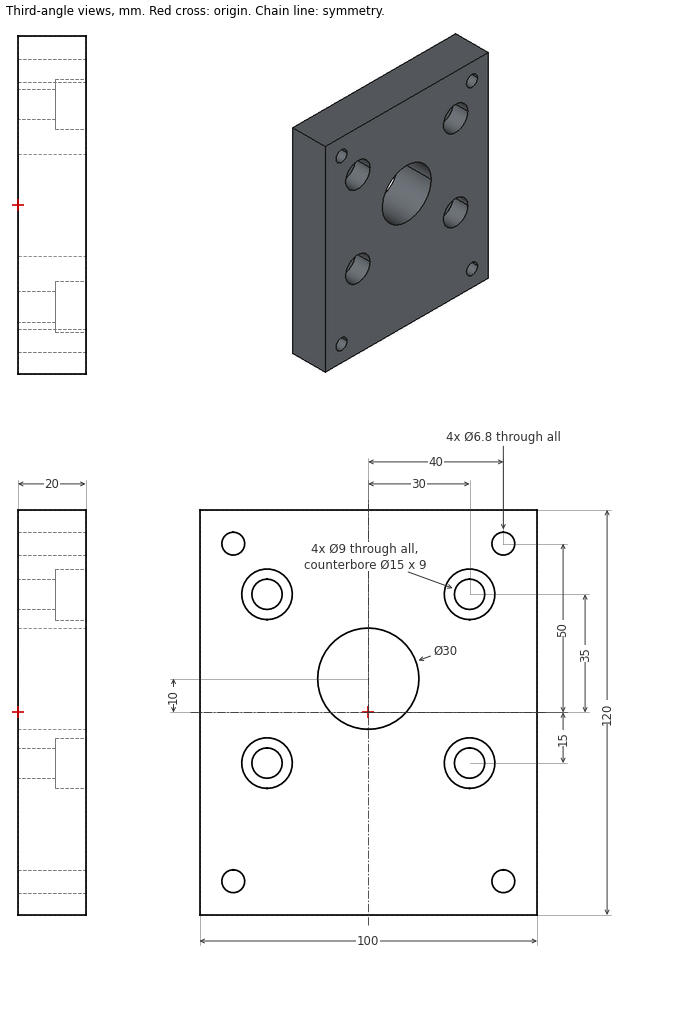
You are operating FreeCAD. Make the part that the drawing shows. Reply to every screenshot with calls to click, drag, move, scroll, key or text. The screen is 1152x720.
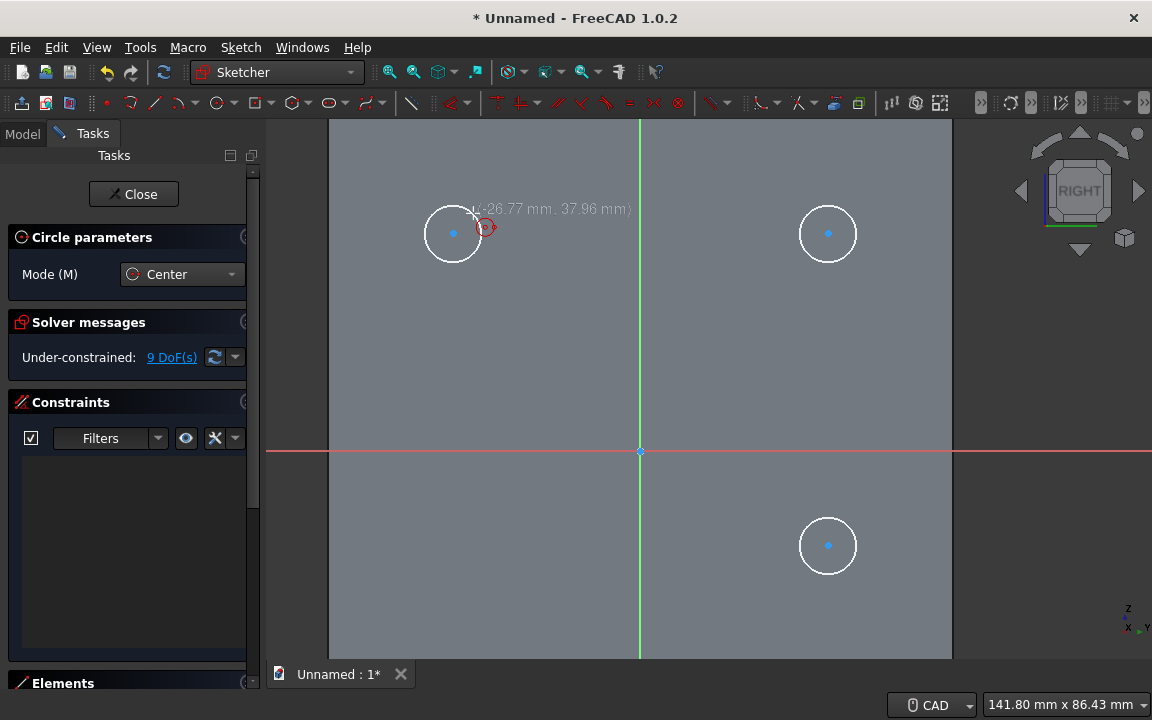
click(453, 545)
click(473, 525)
key(Escape)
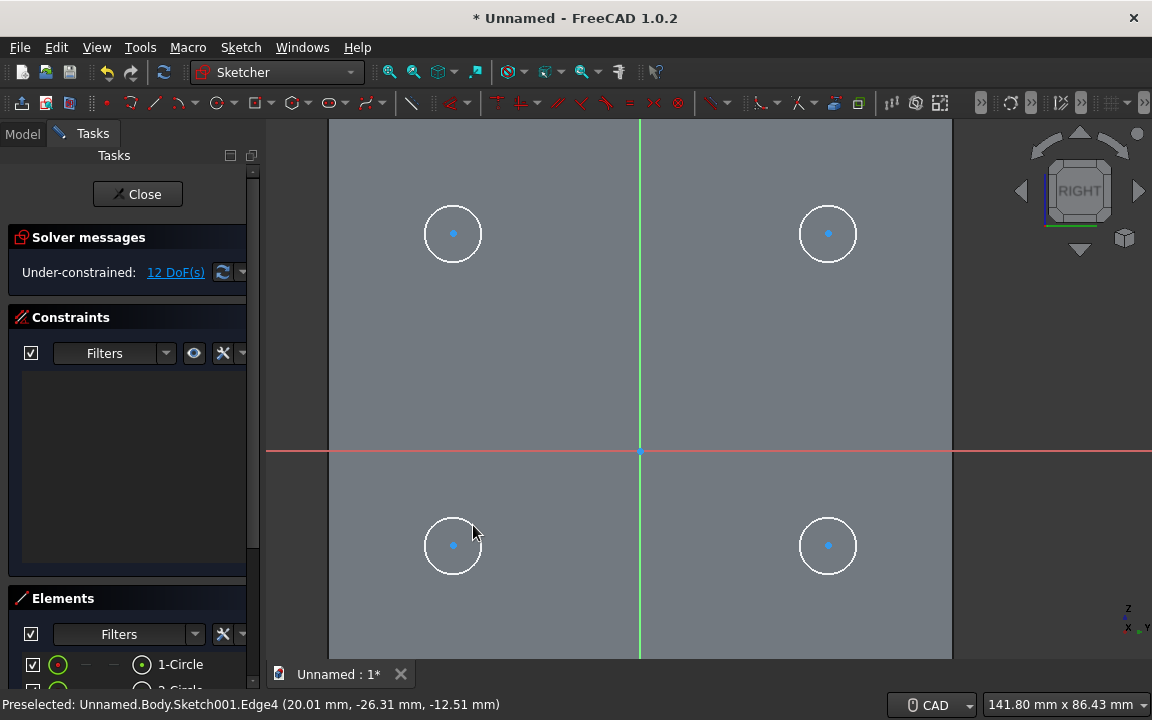
click(848, 214)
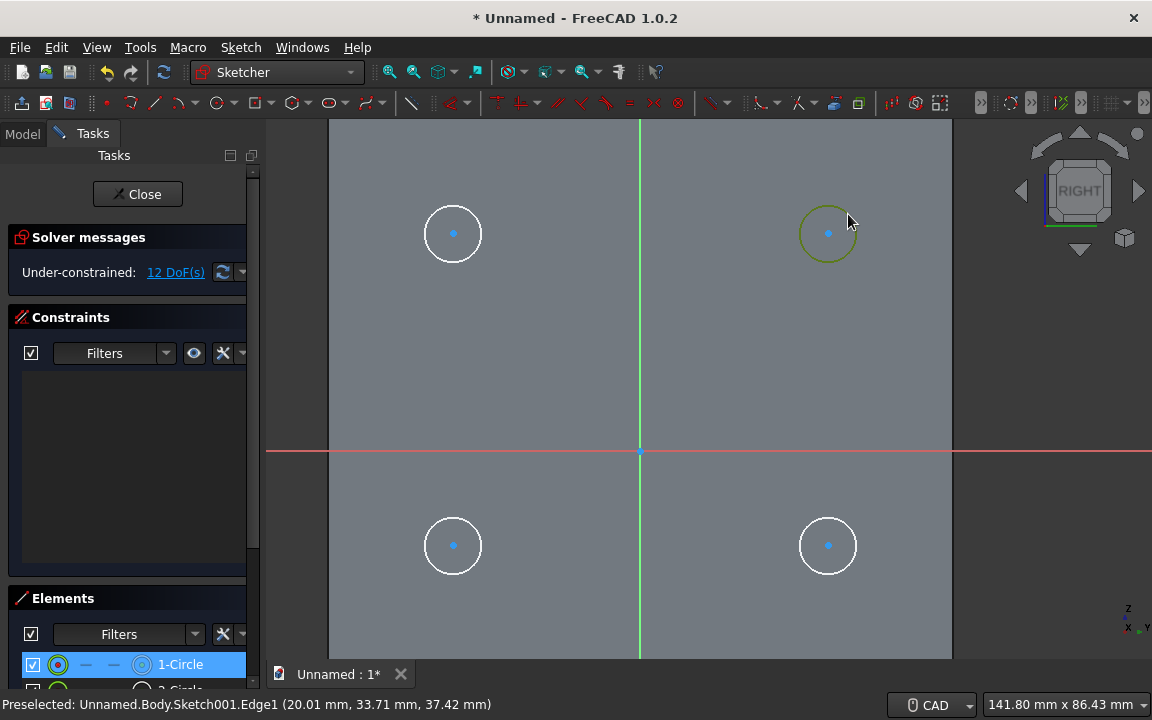
click(848, 526)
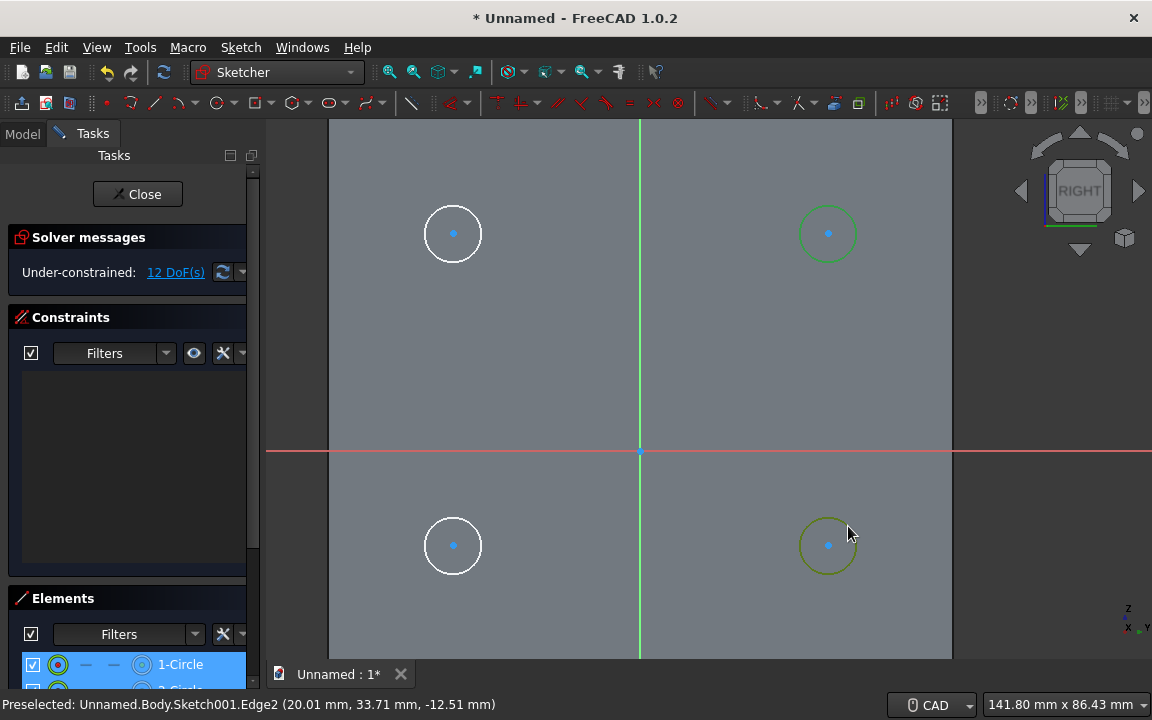
click(473, 214)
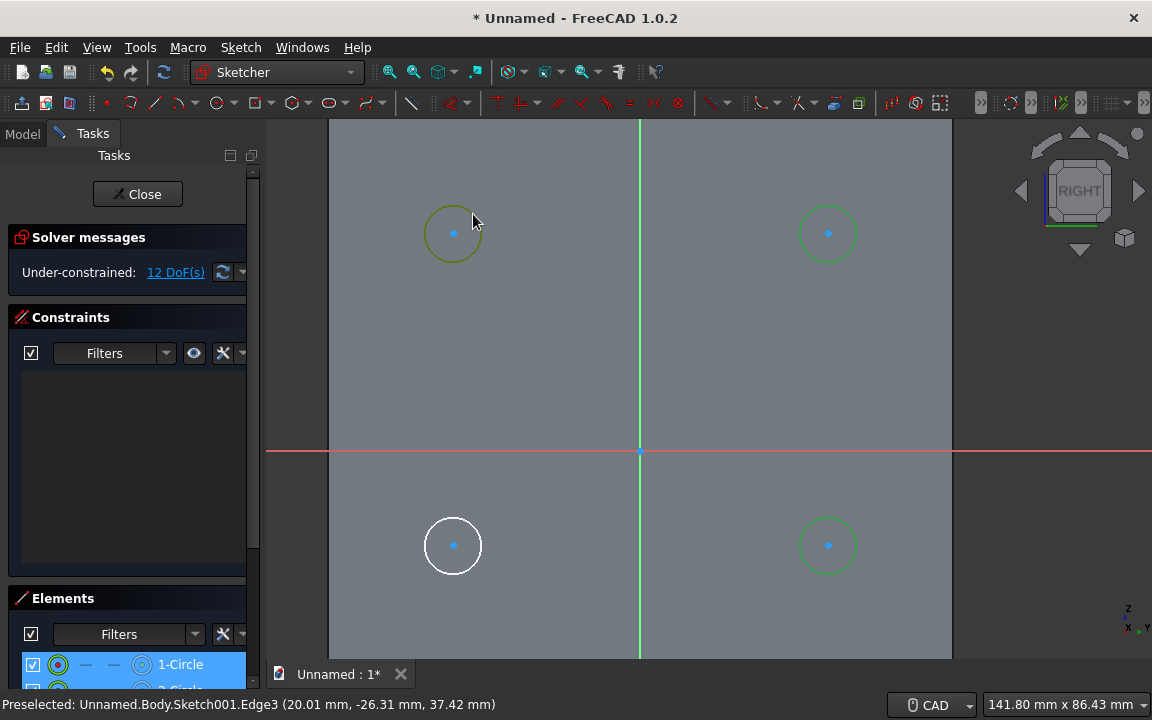
click(473, 526)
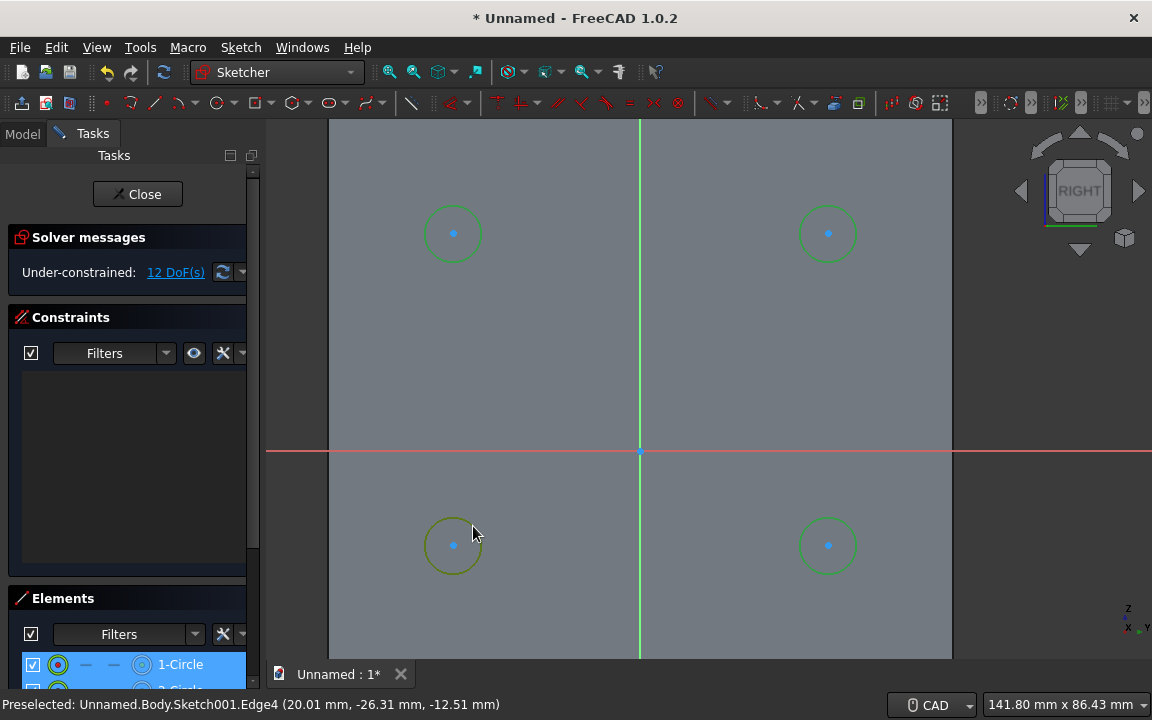
click(630, 104)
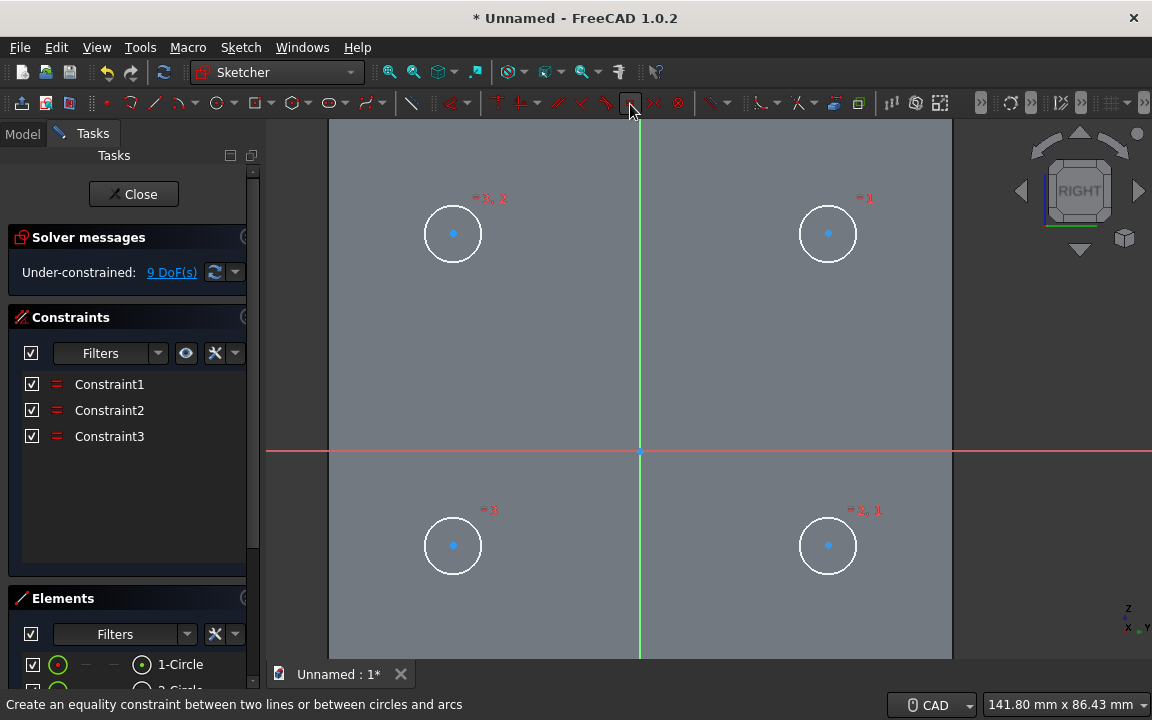
click(828, 234)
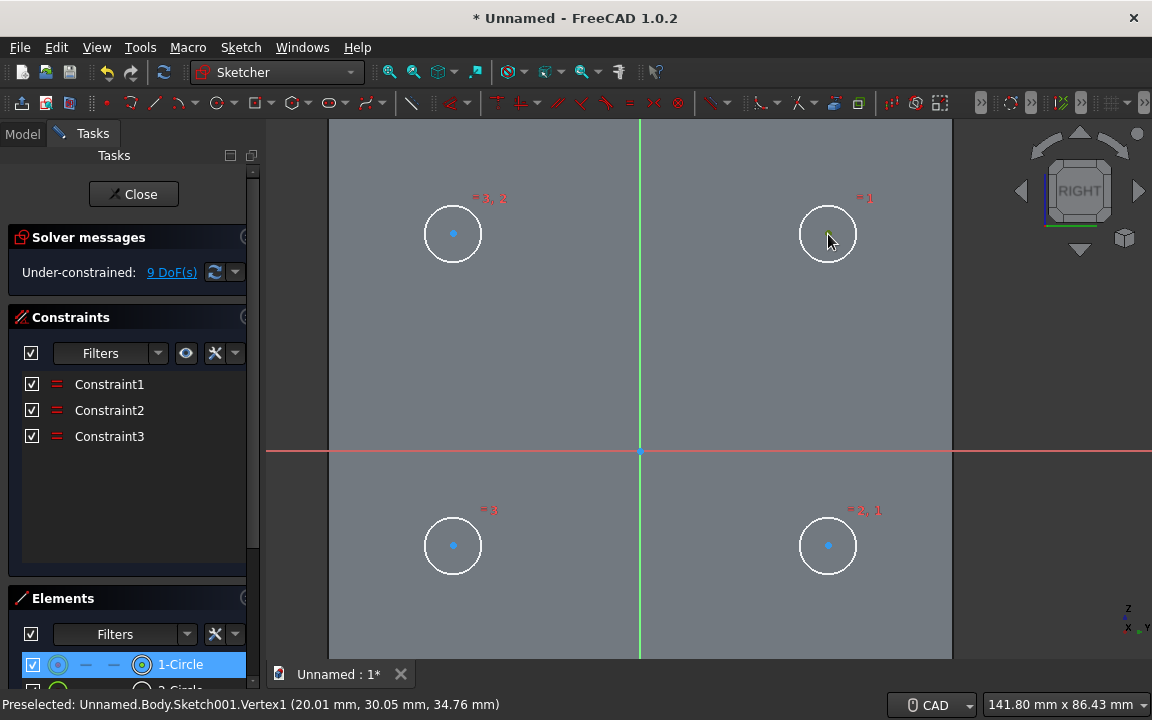
click(453, 234)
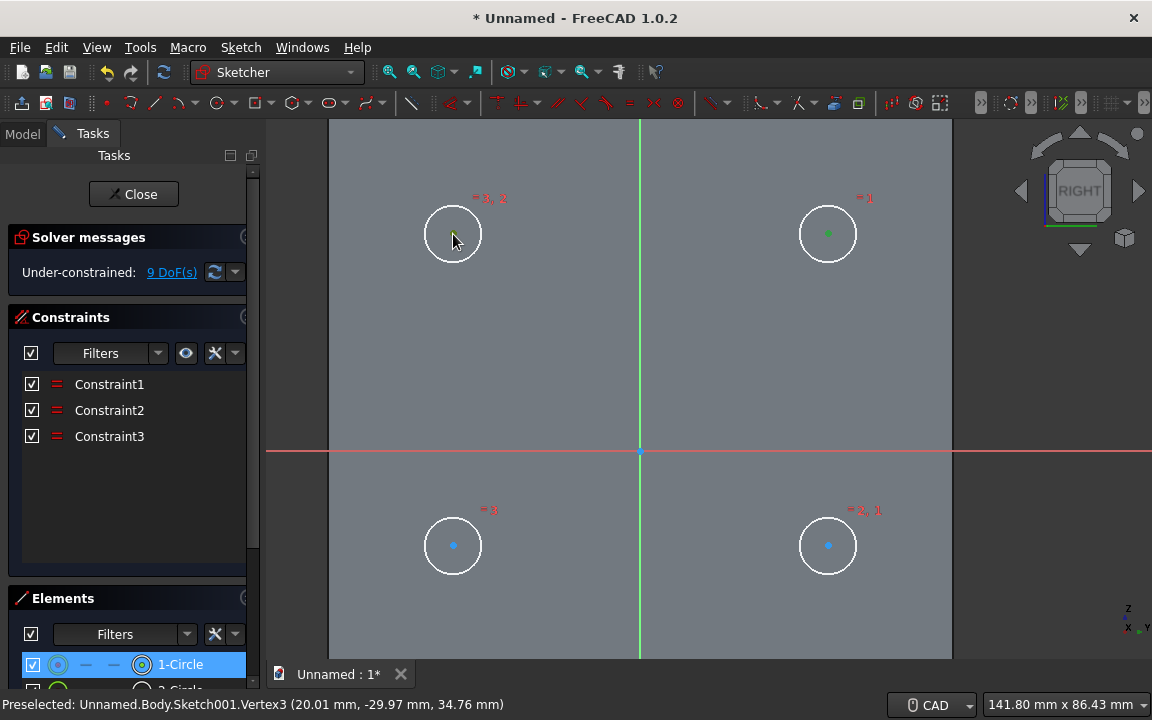
click(640, 596)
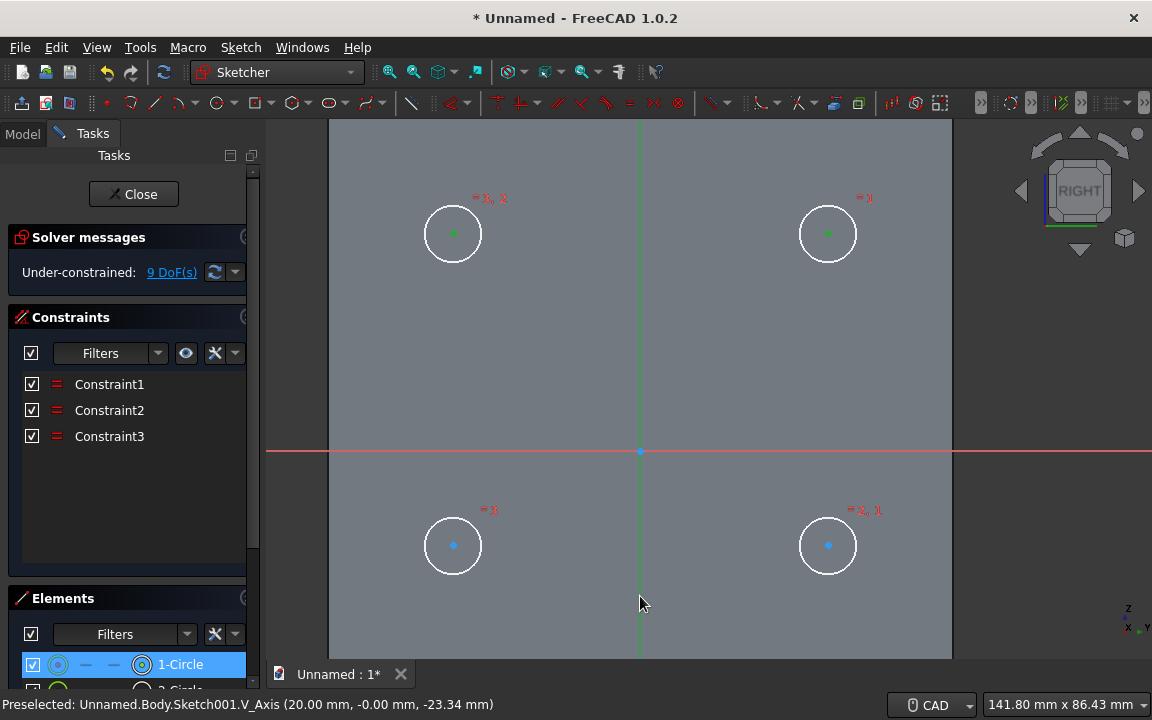
click(654, 104)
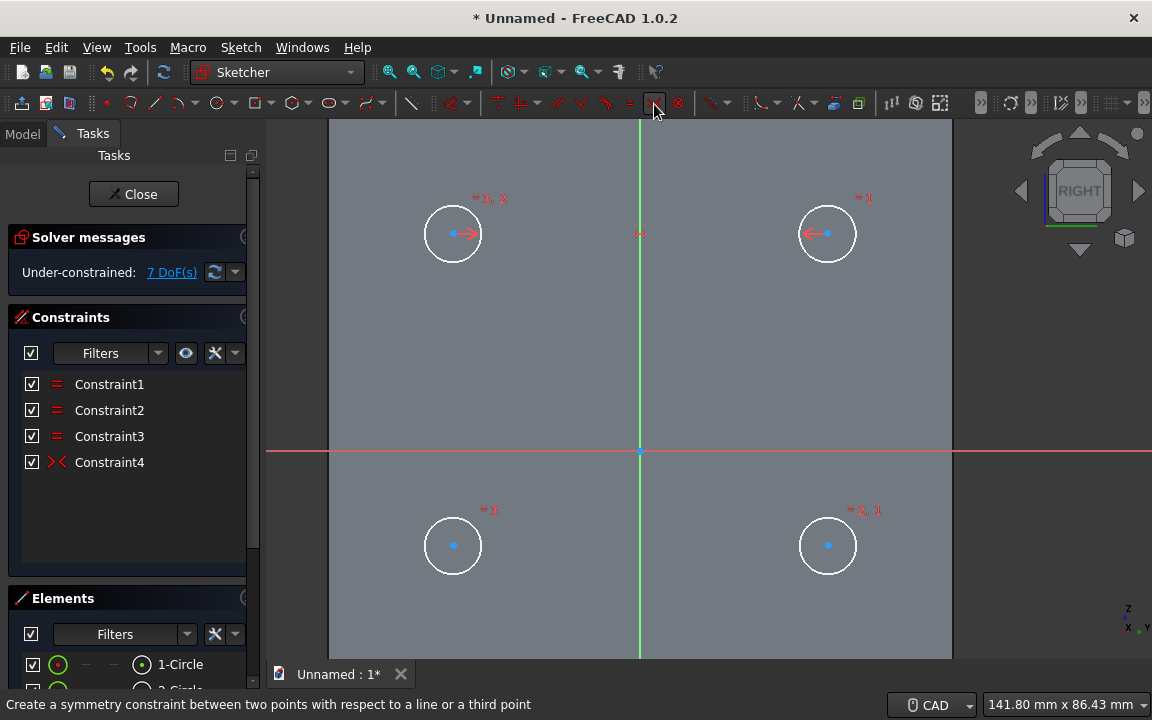
click(828, 546)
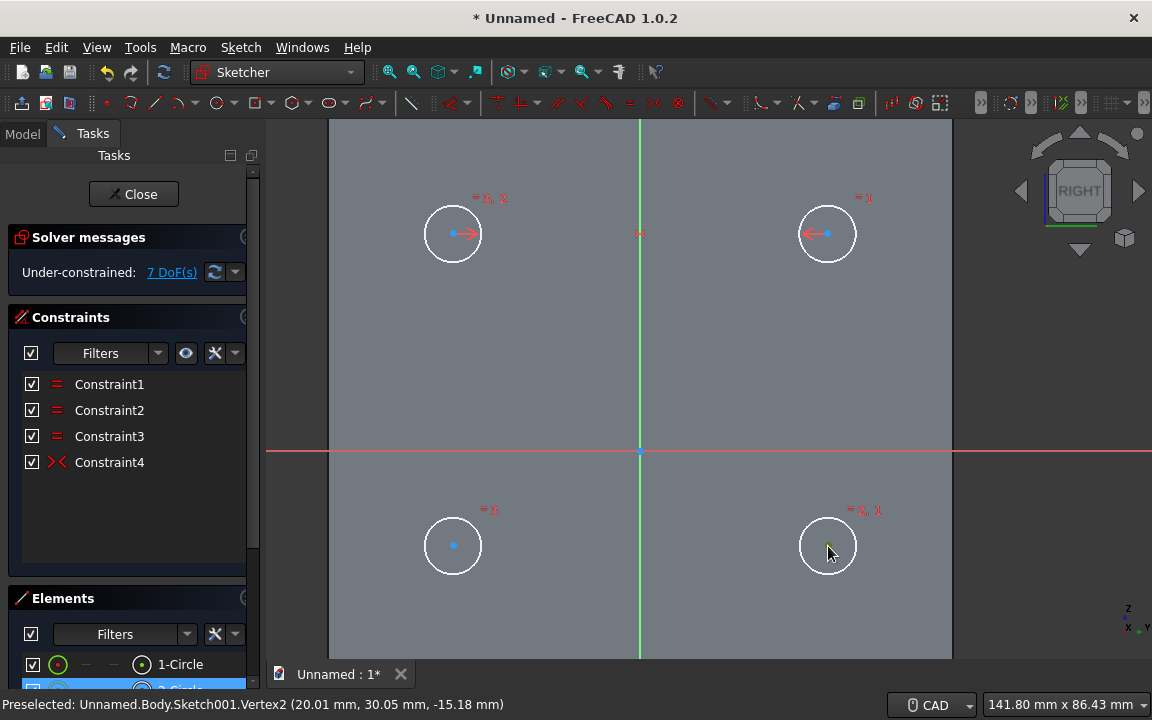
click(453, 546)